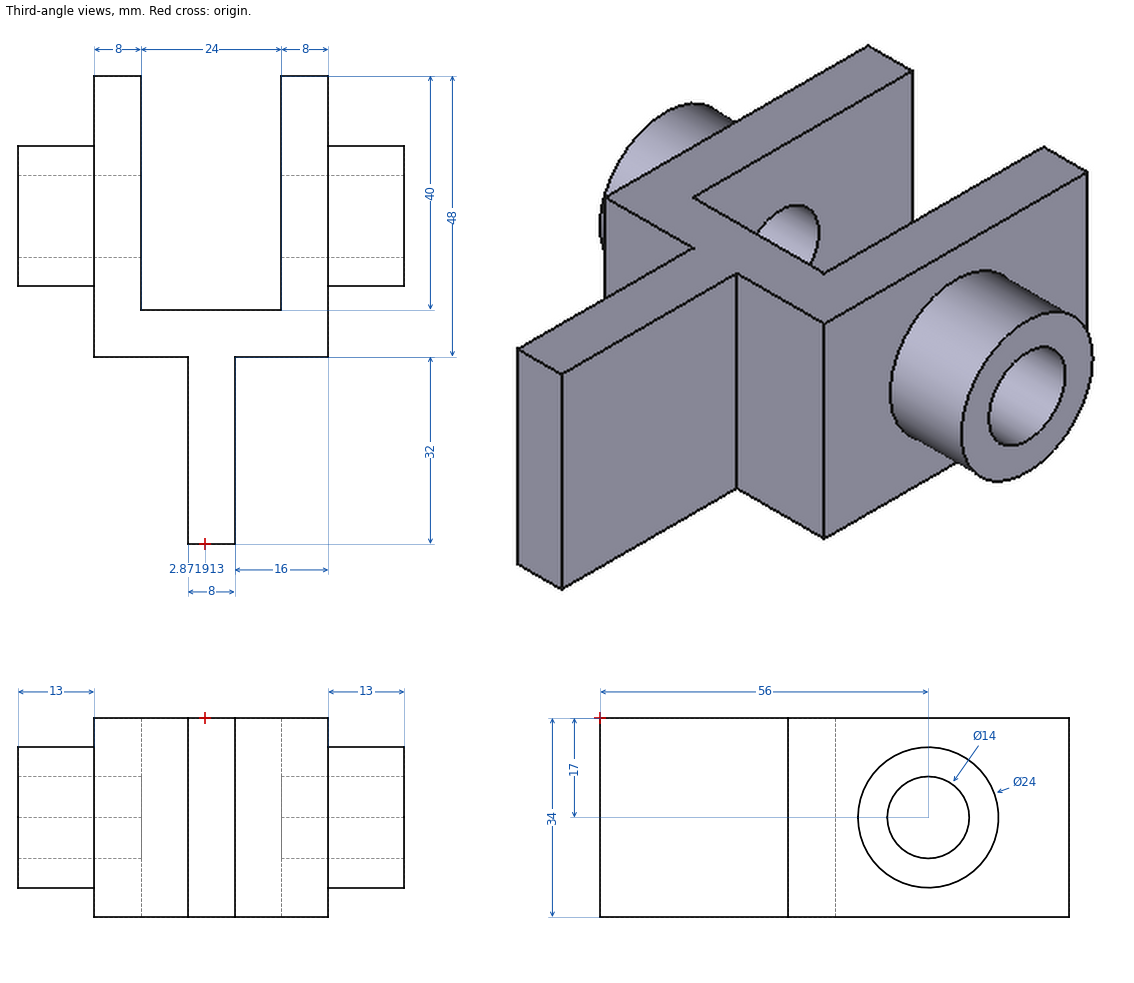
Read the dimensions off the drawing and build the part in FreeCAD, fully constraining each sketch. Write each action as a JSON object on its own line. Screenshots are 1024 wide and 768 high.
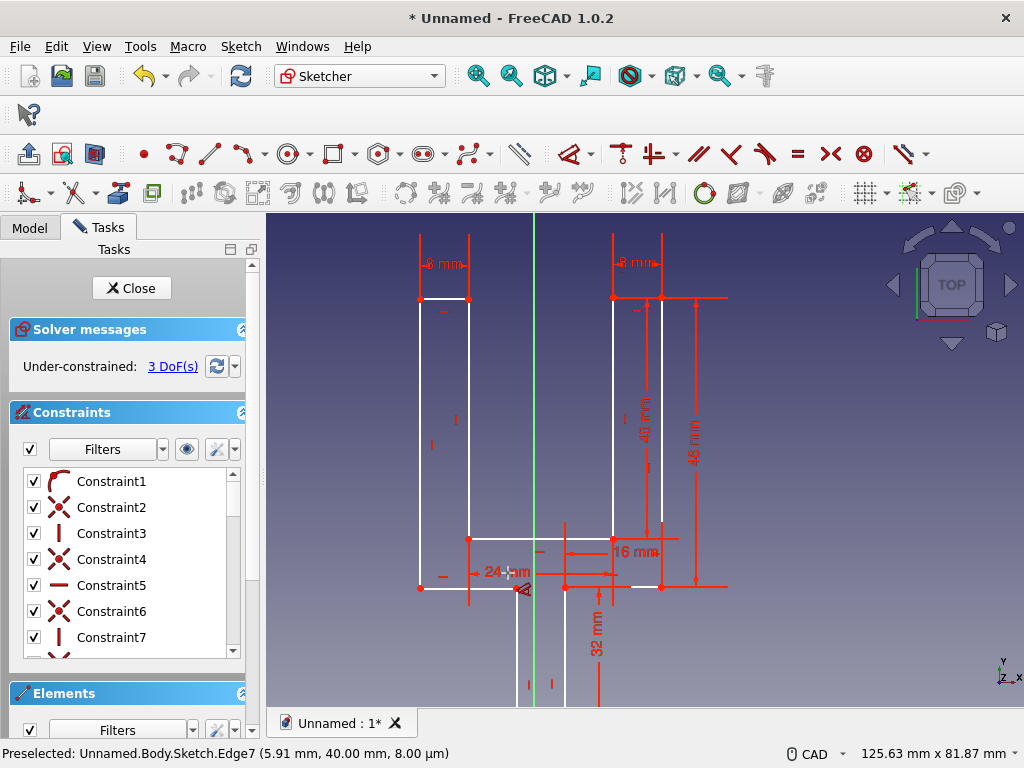
{"action": "left_click", "coordinate": [469, 467]}
{"action": "left_click", "coordinate": [435, 419]}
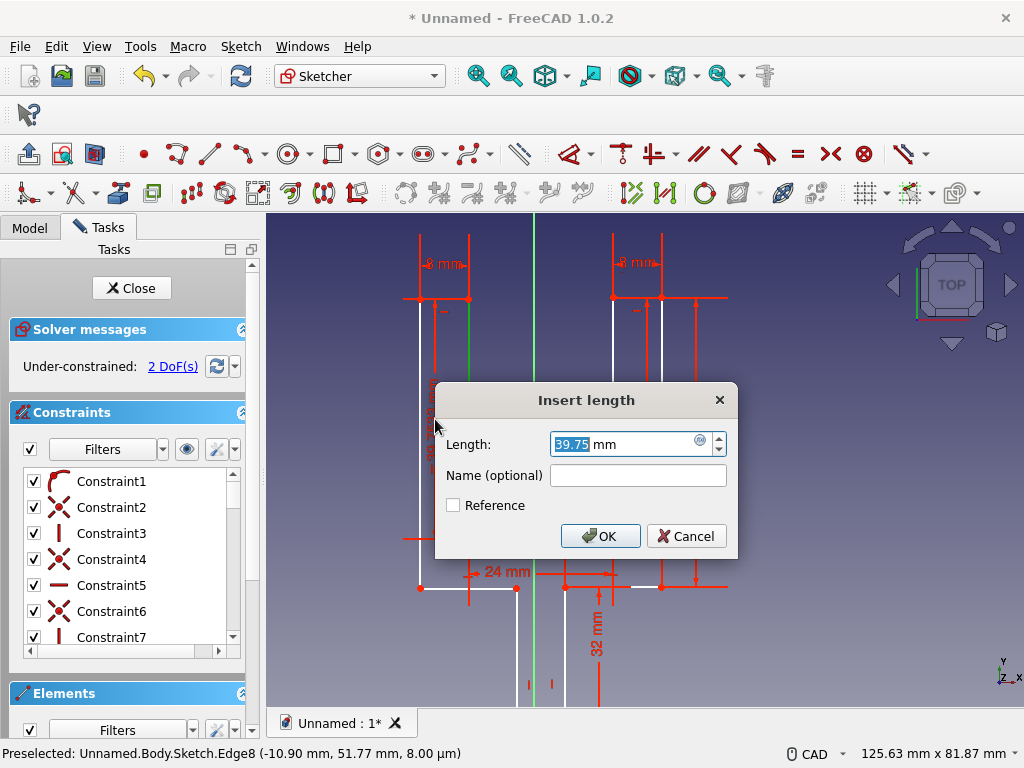
{"action": "type", "text": "40"}
{"action": "key", "text": "Return"}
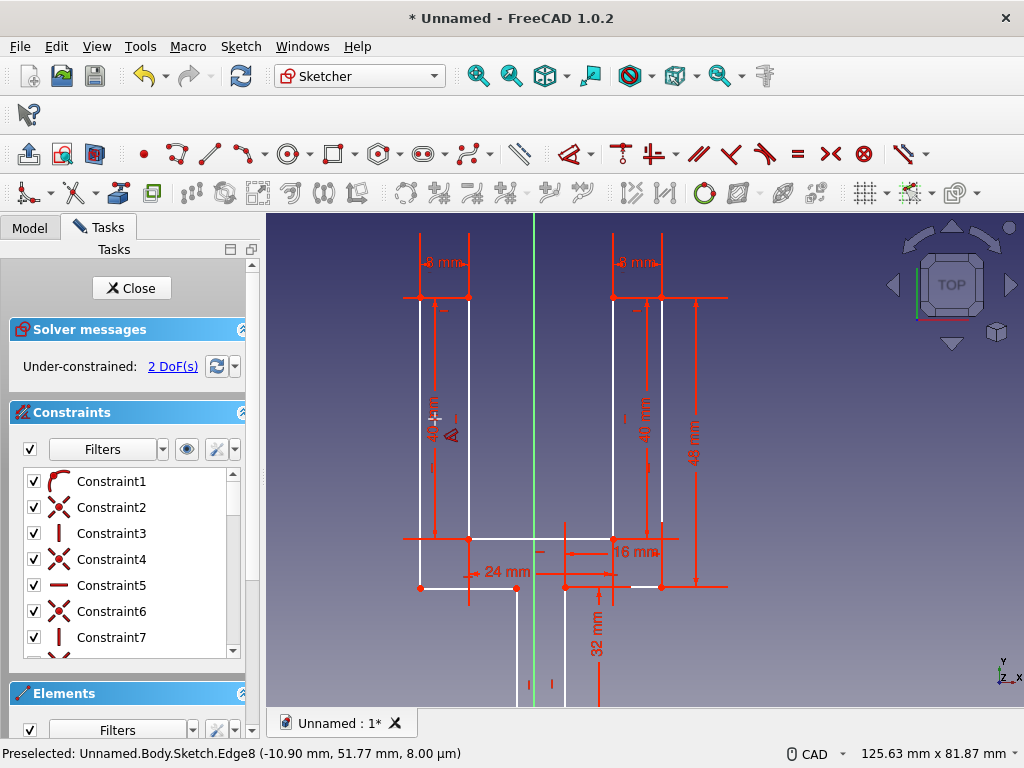
{"action": "left_click", "coordinate": [420, 385]}
{"action": "left_click", "coordinate": [386, 443]}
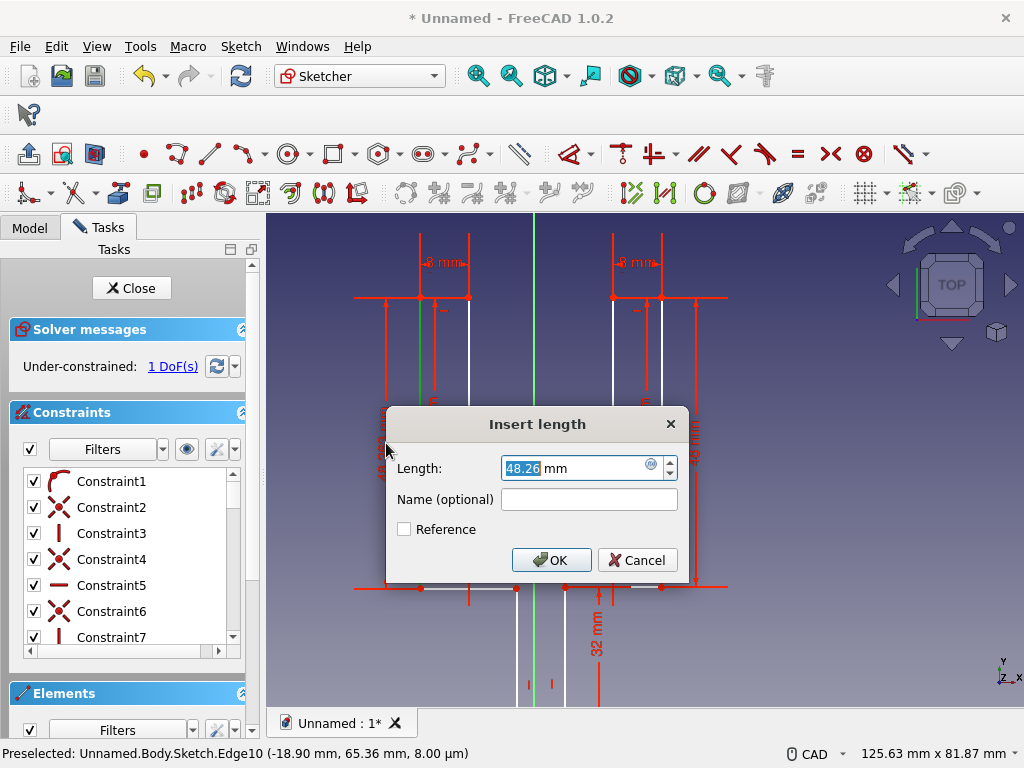
{"action": "type", "text": "48"}
{"action": "key", "text": "Return"}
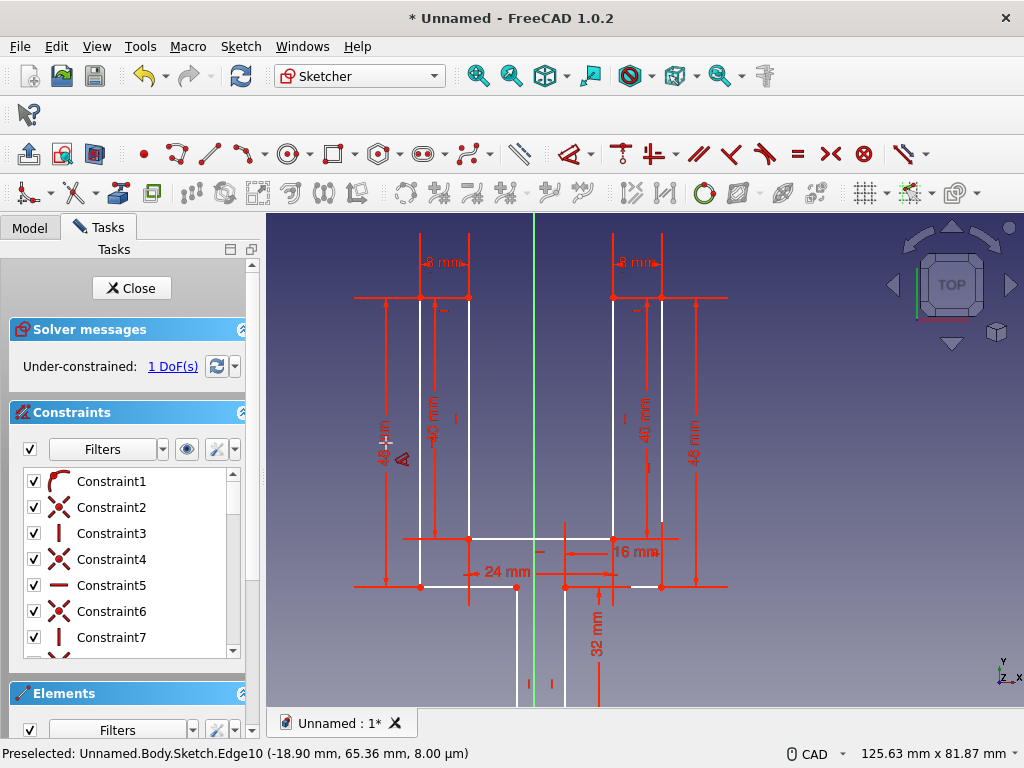
{"action": "scroll", "coordinate": [648, 299], "scroll_direction": "down", "scroll_amount": 2}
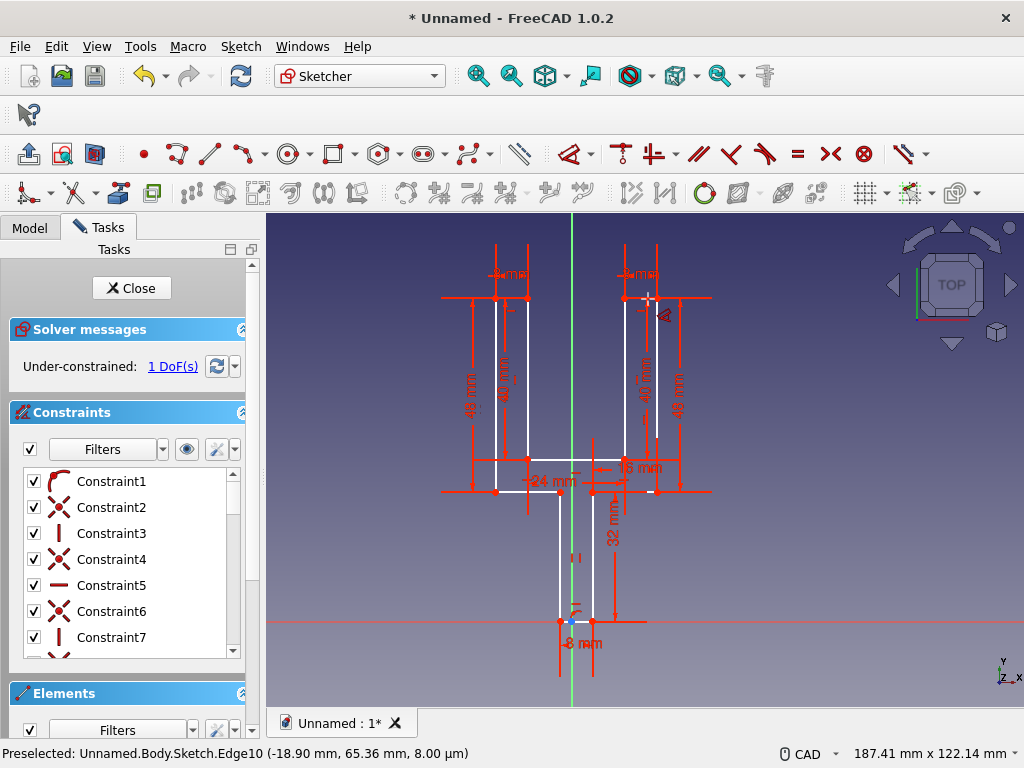
{"action": "scroll", "coordinate": [560, 622], "scroll_direction": "up", "scroll_amount": 7}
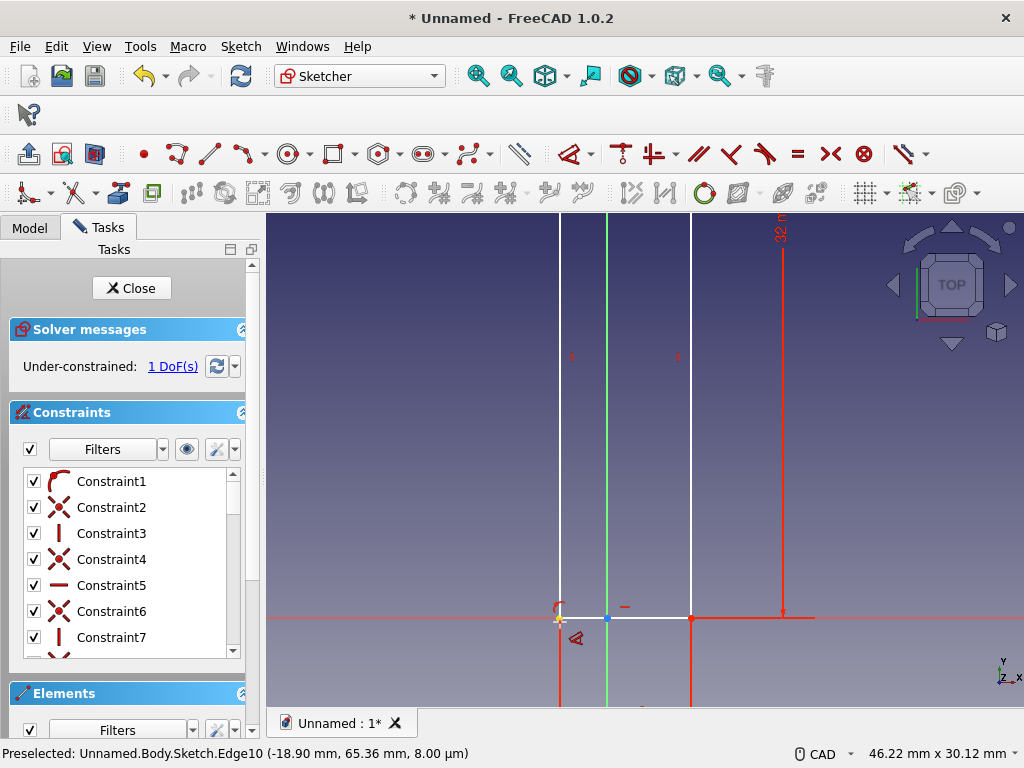
{"action": "left_click", "coordinate": [560, 618]}
{"action": "left_click", "coordinate": [584, 652]}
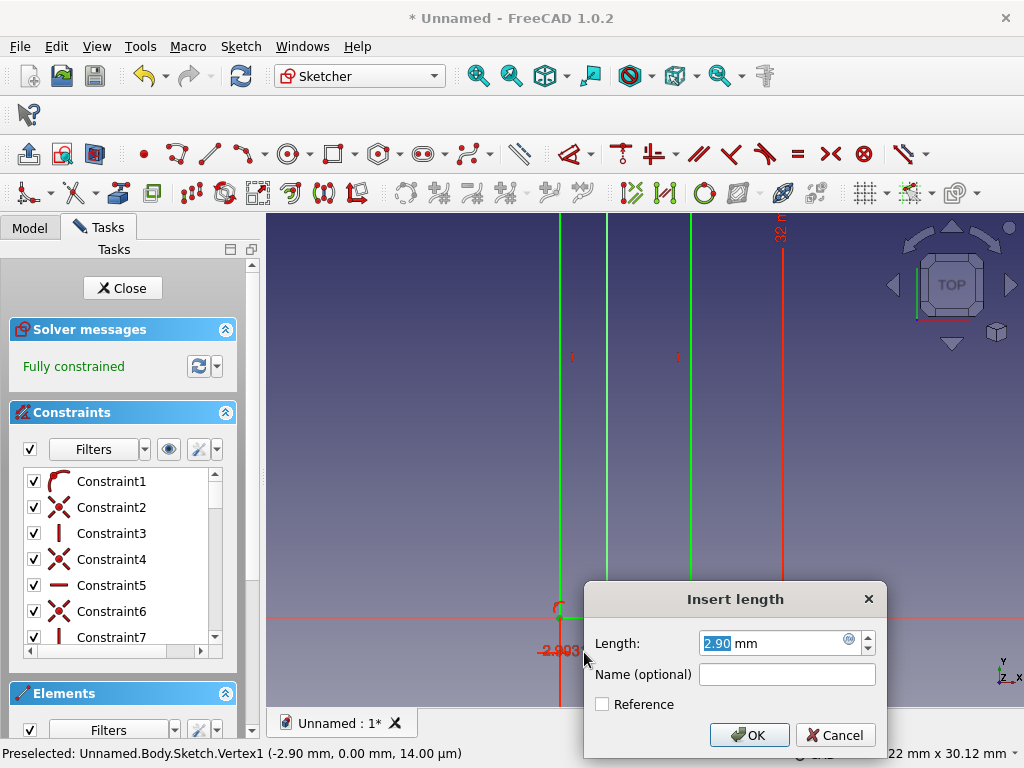
{"action": "type", "text": "2.871913"}
{"action": "key", "text": "Return"}
{"action": "key", "text": "Escape"}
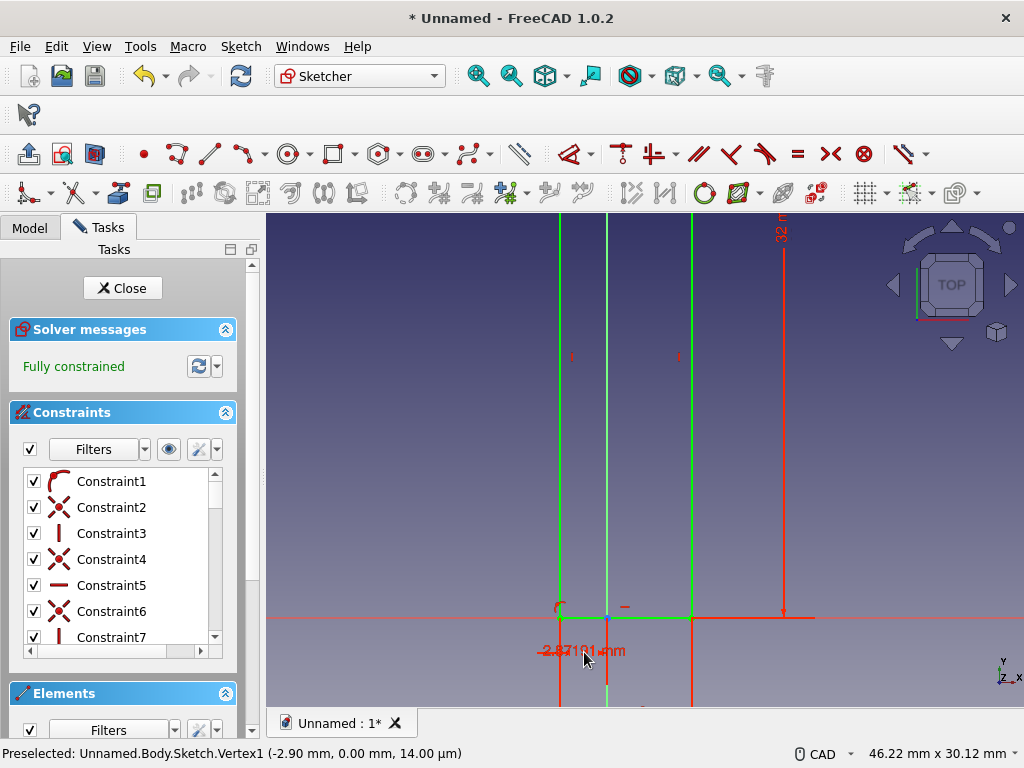
{"action": "left_click", "coordinate": [123, 288]}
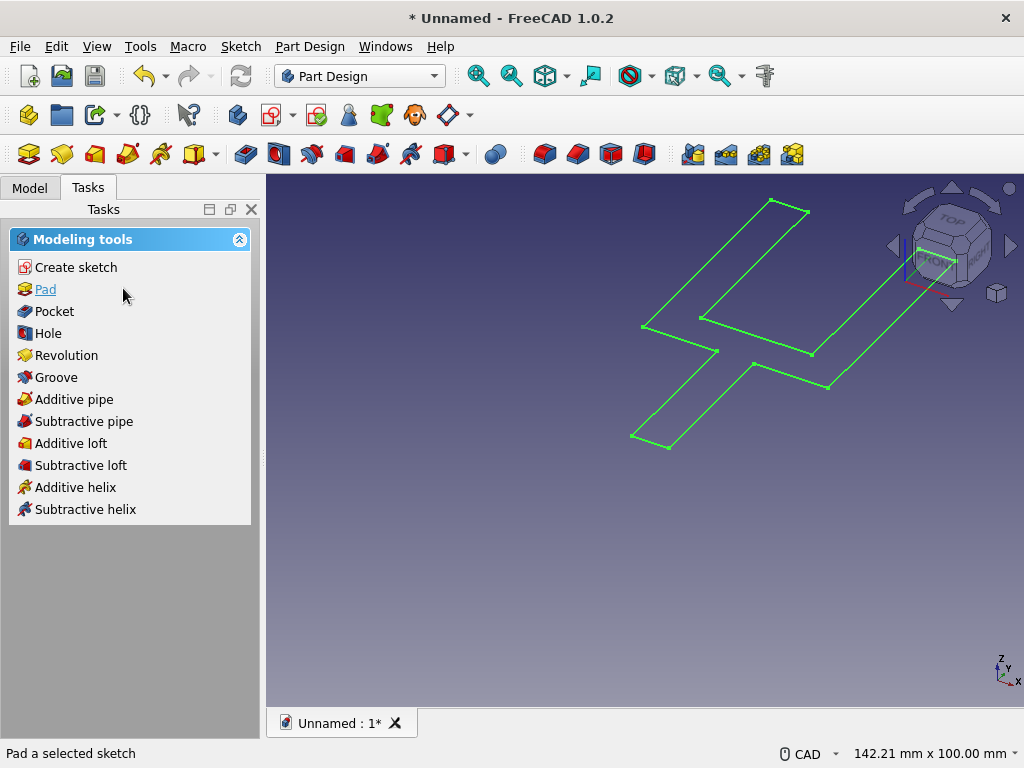
{"action": "left_click", "coordinate": [29, 154]}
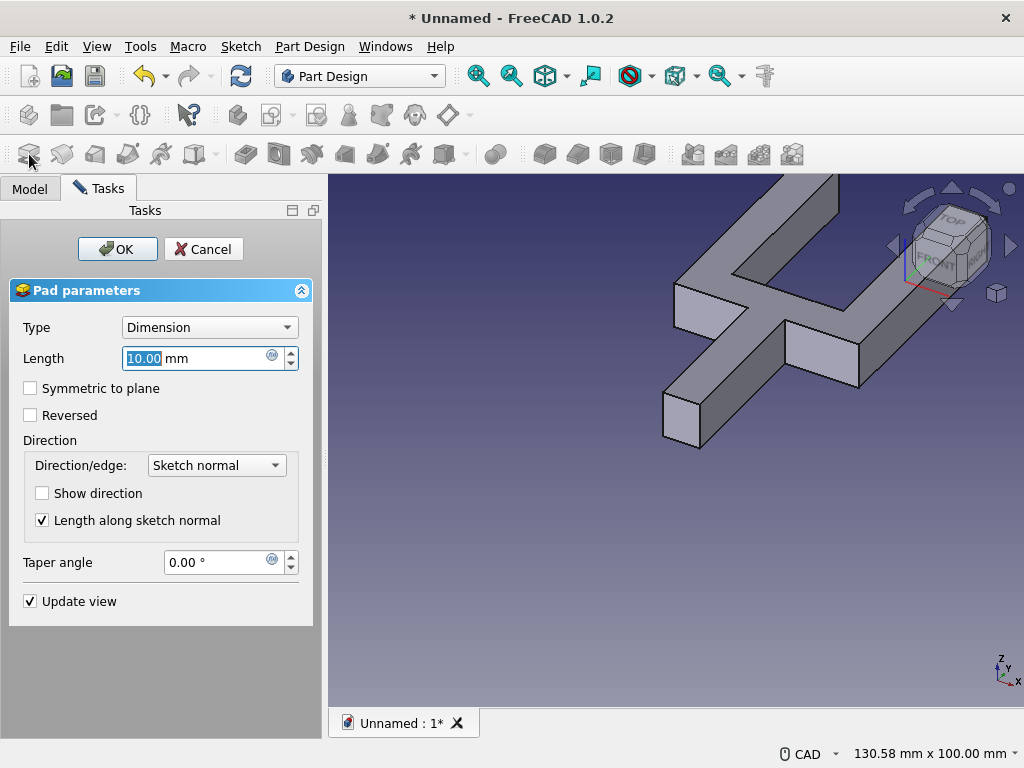
{"action": "type", "text": "34"}
{"action": "key", "text": "Tab"}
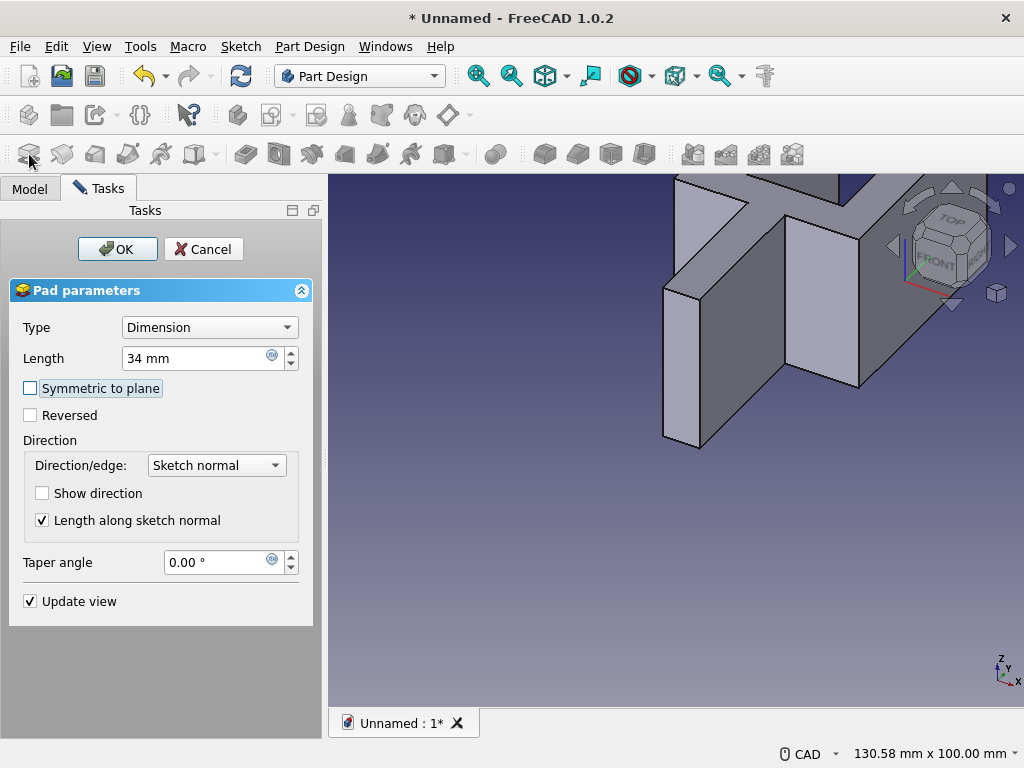
{"action": "left_click", "coordinate": [31, 415]}